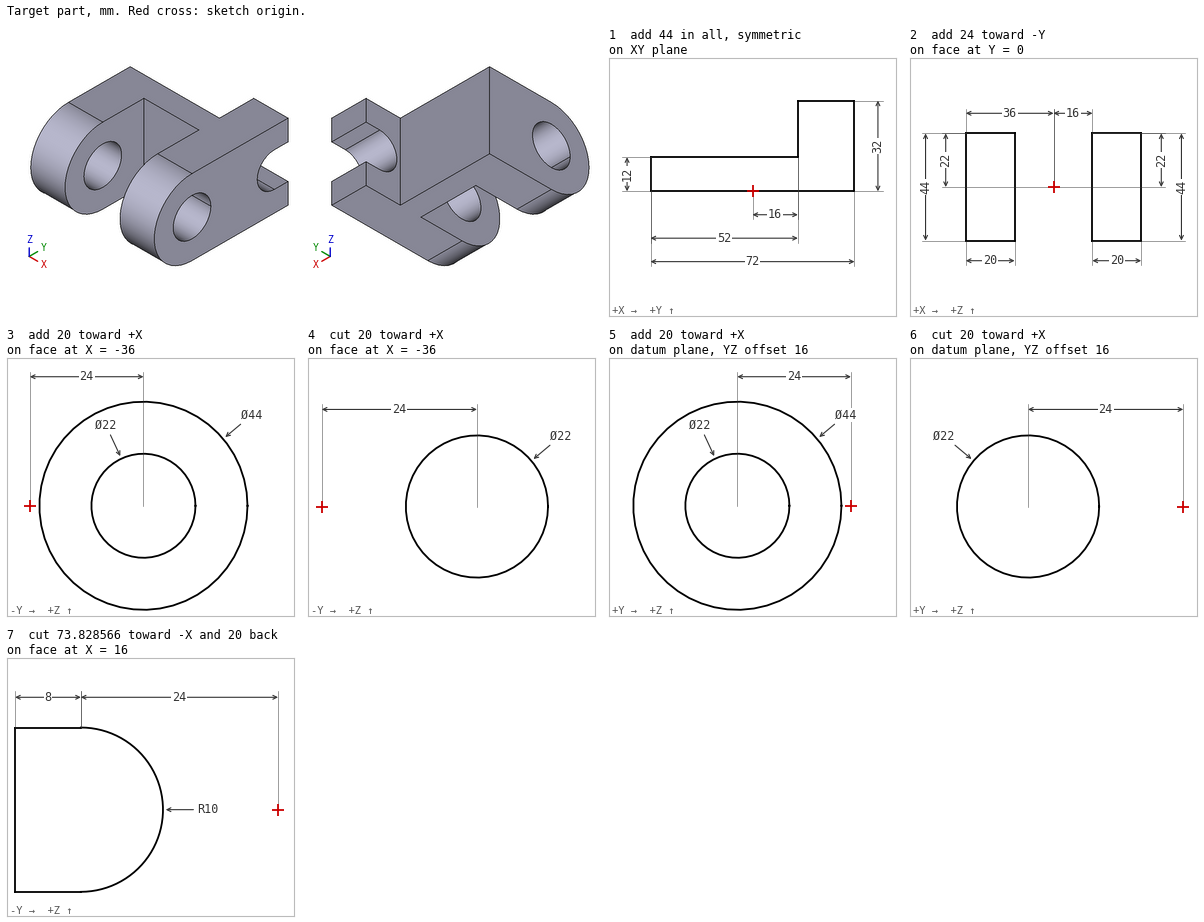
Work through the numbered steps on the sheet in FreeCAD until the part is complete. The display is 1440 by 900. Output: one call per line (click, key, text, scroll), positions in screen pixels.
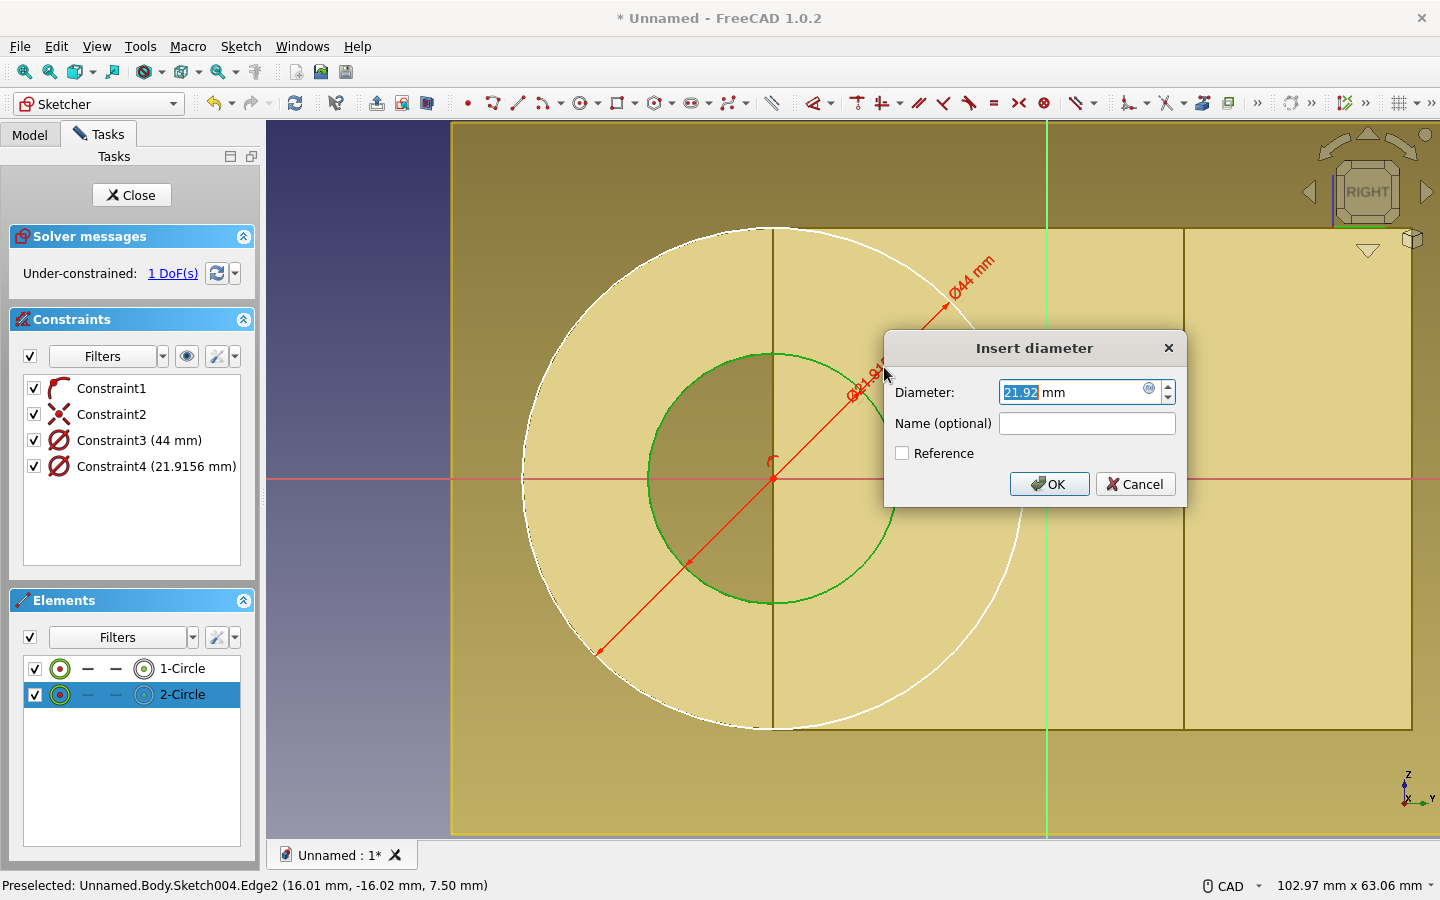
text(22)
key(Return)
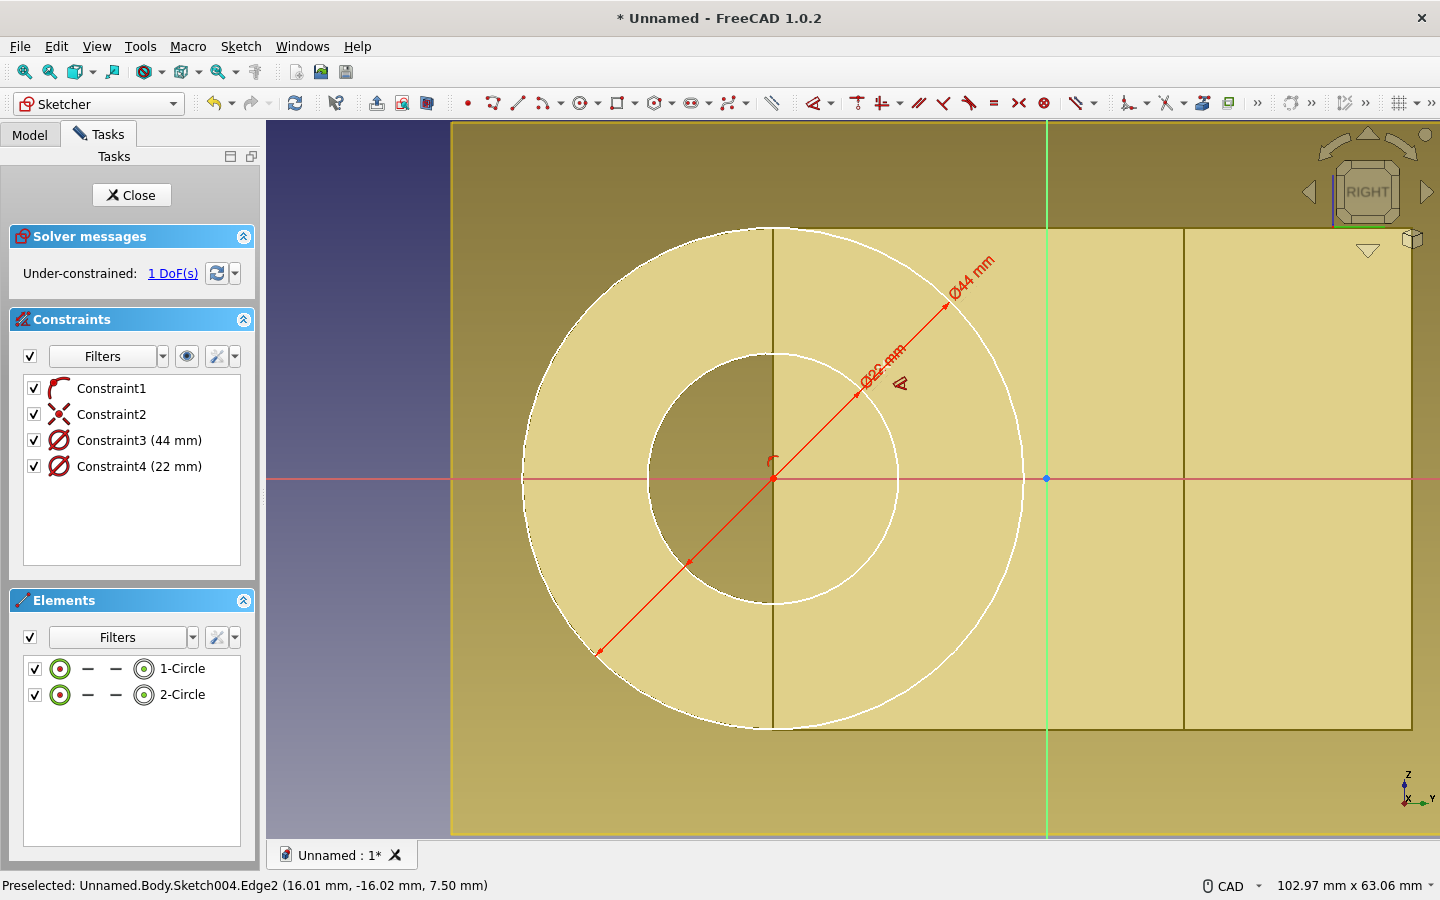
click(773, 479)
click(910, 513)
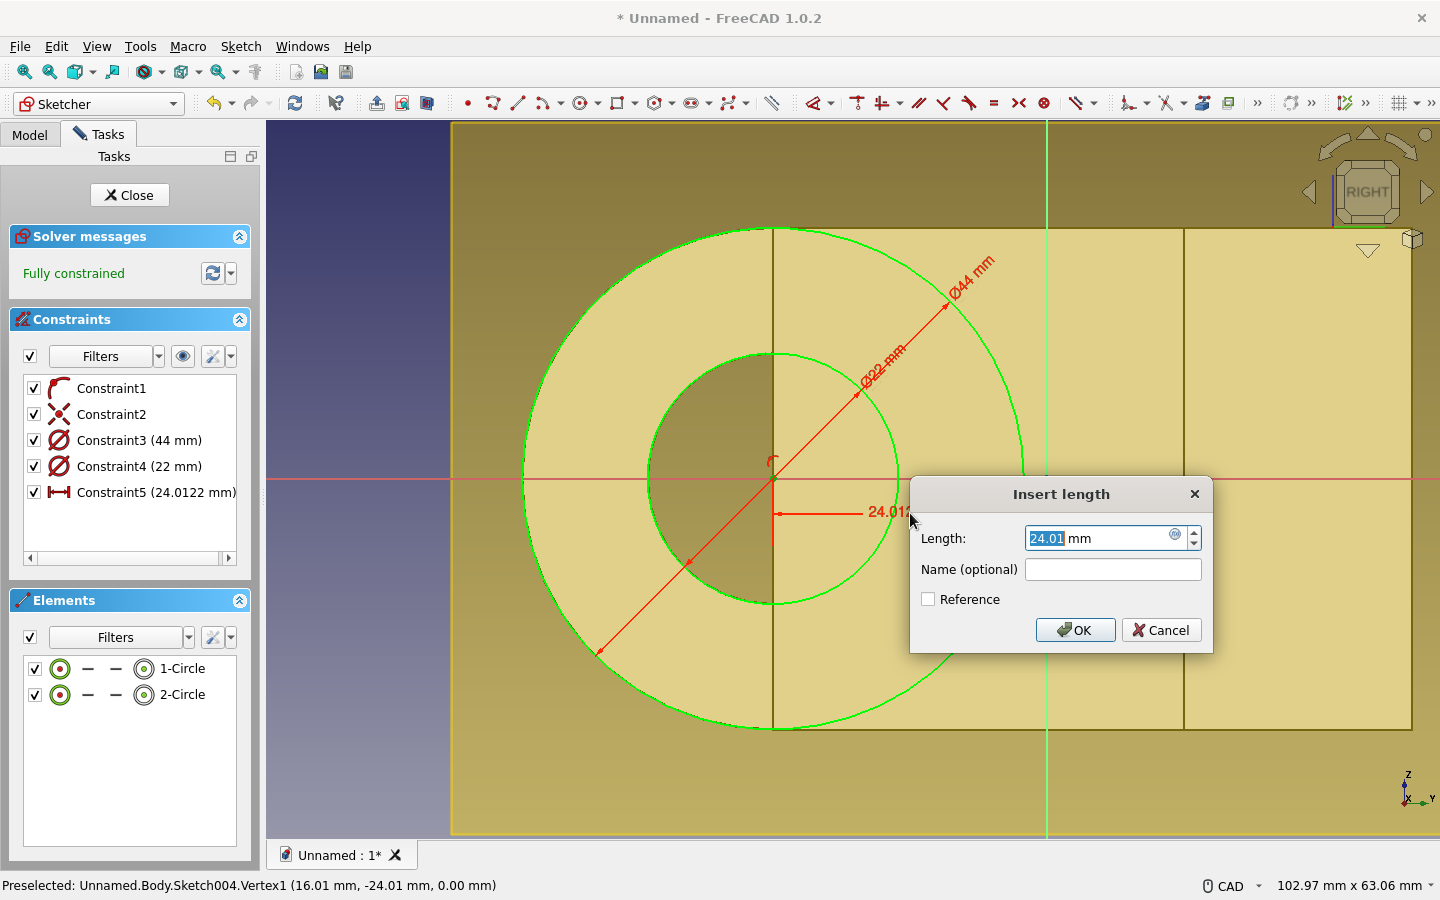
text(24)
key(Return)
key(Escape)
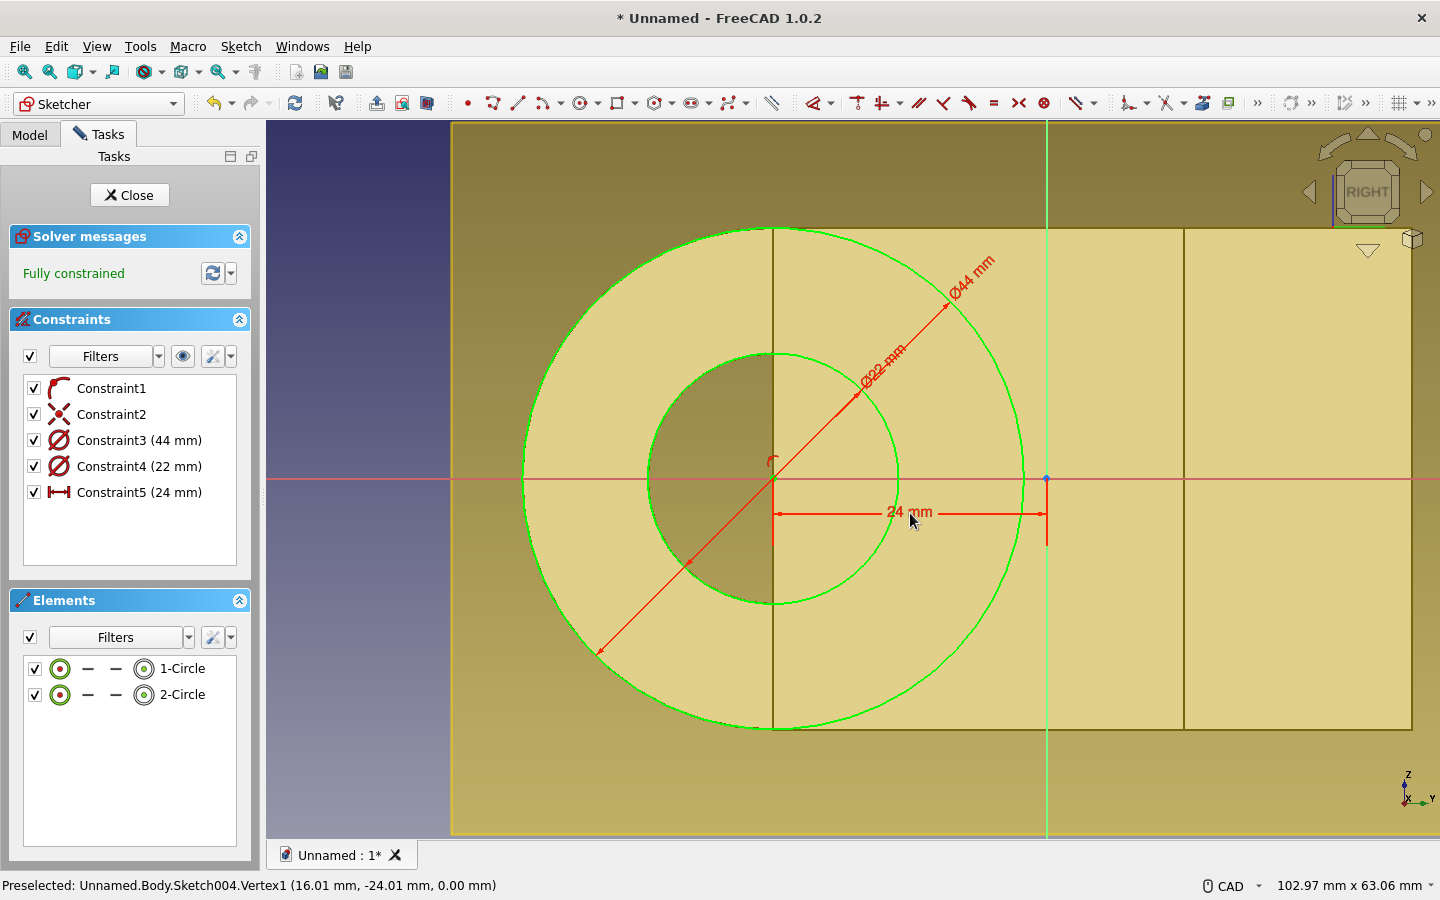
click(130, 195)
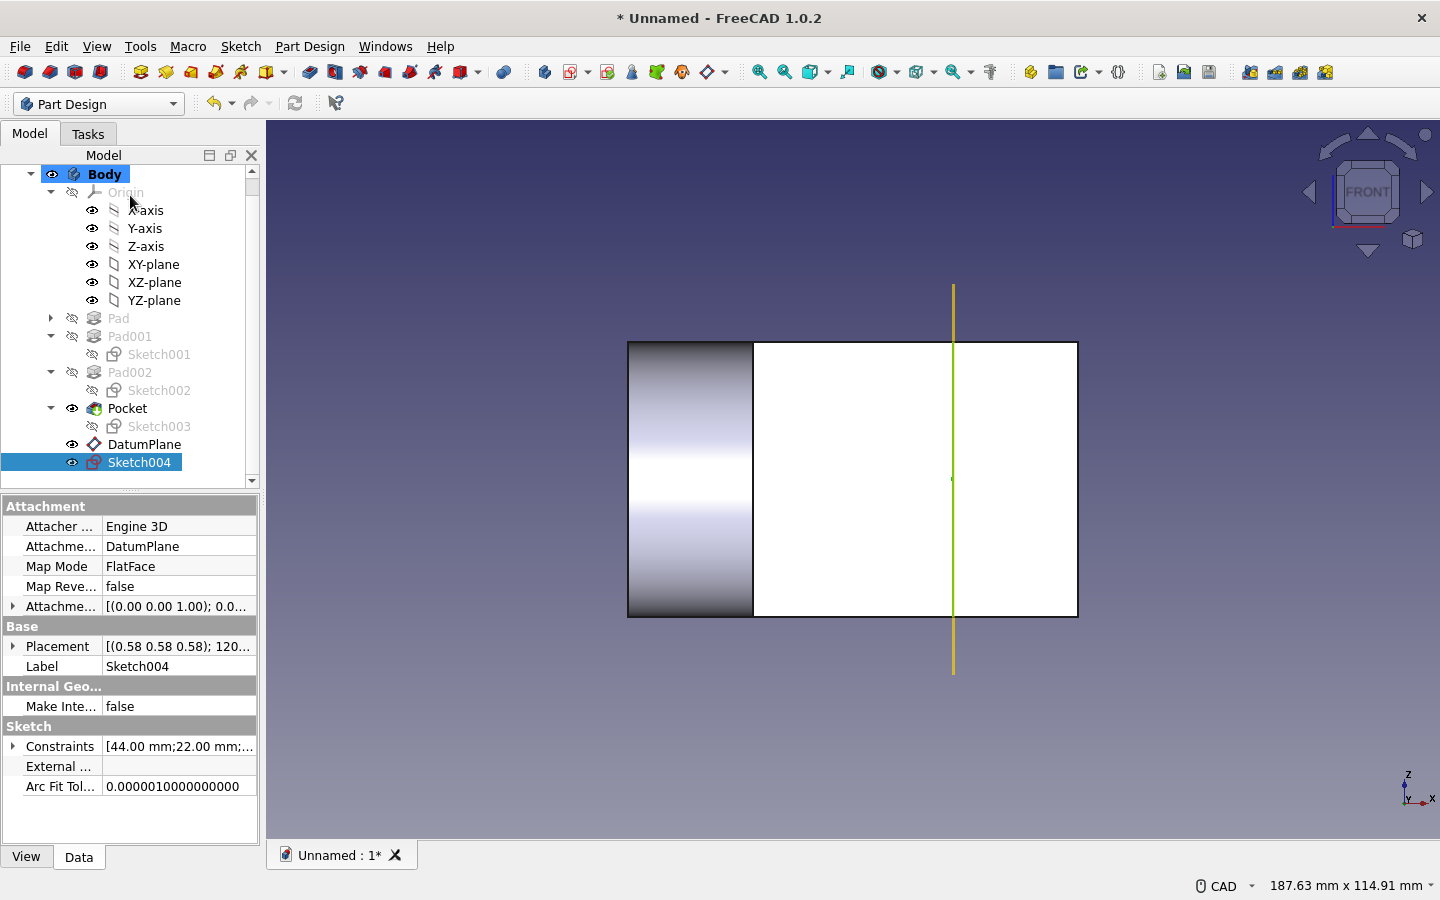
click(141, 72)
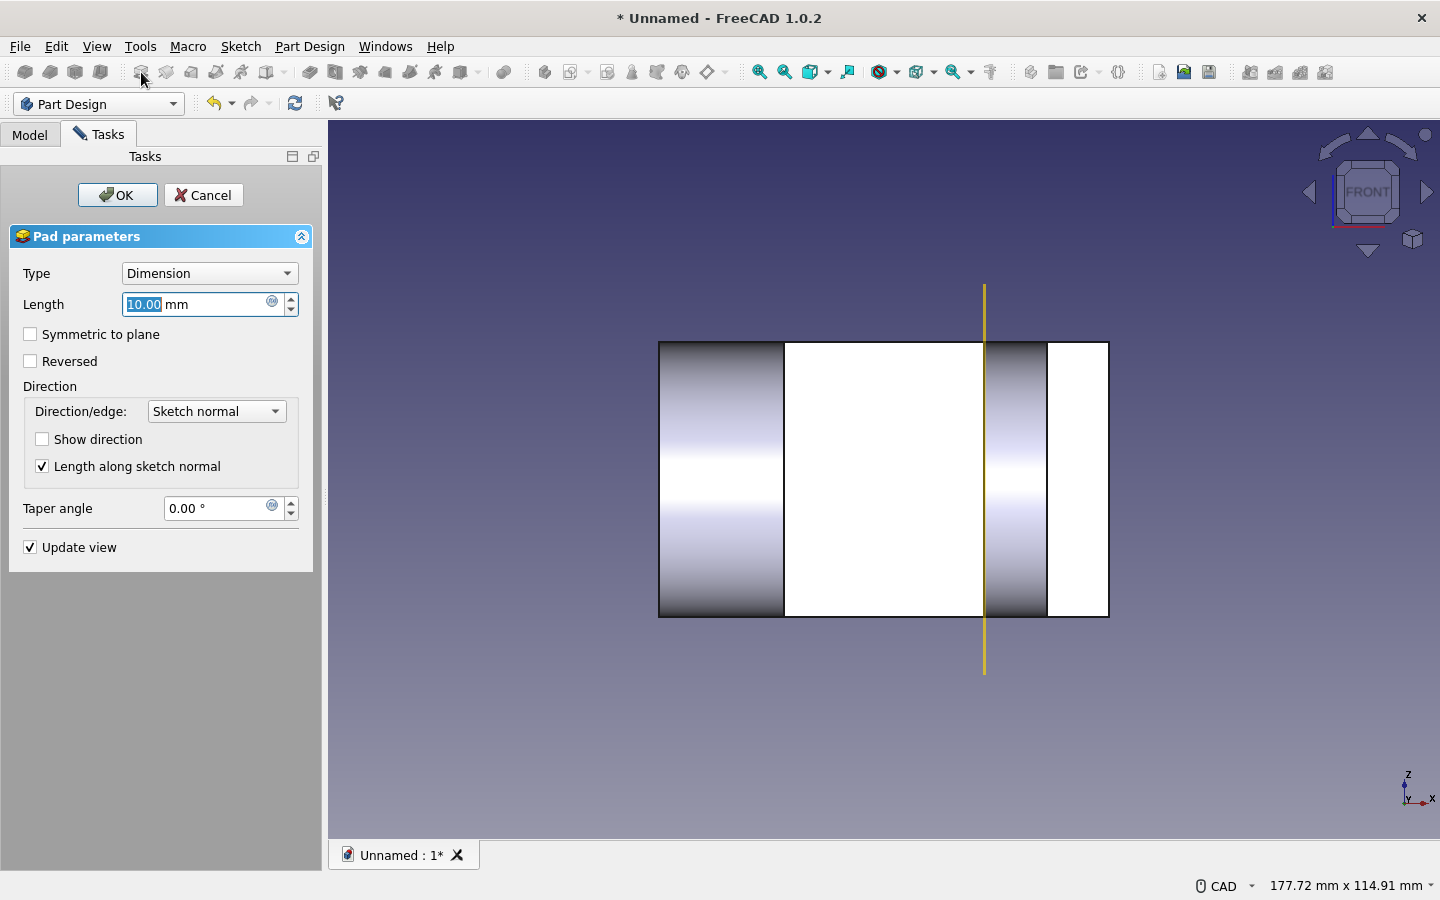
text(20)
key(Tab)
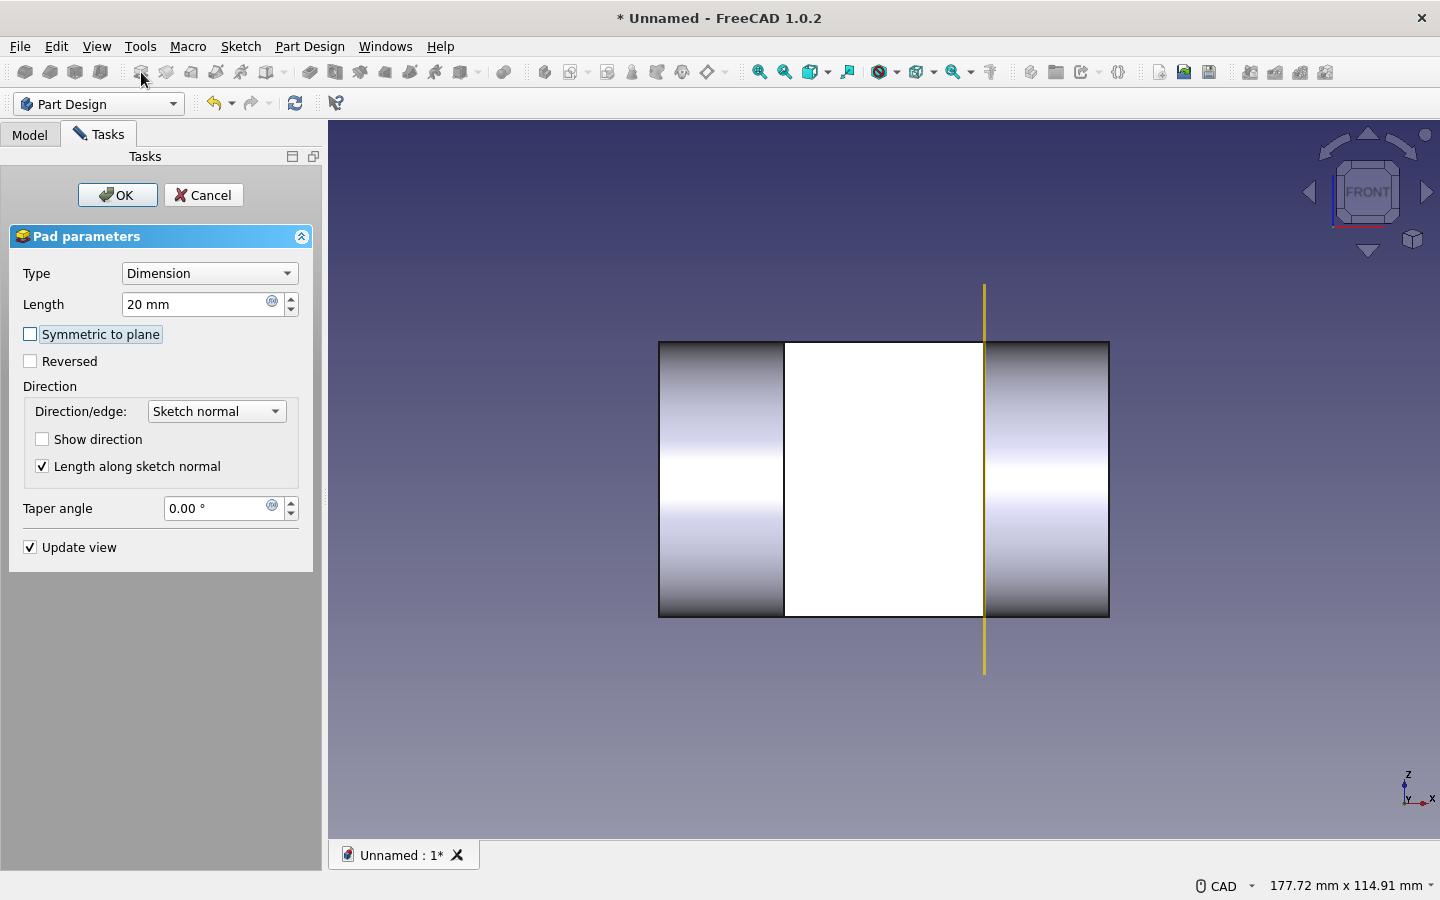
click(118, 195)